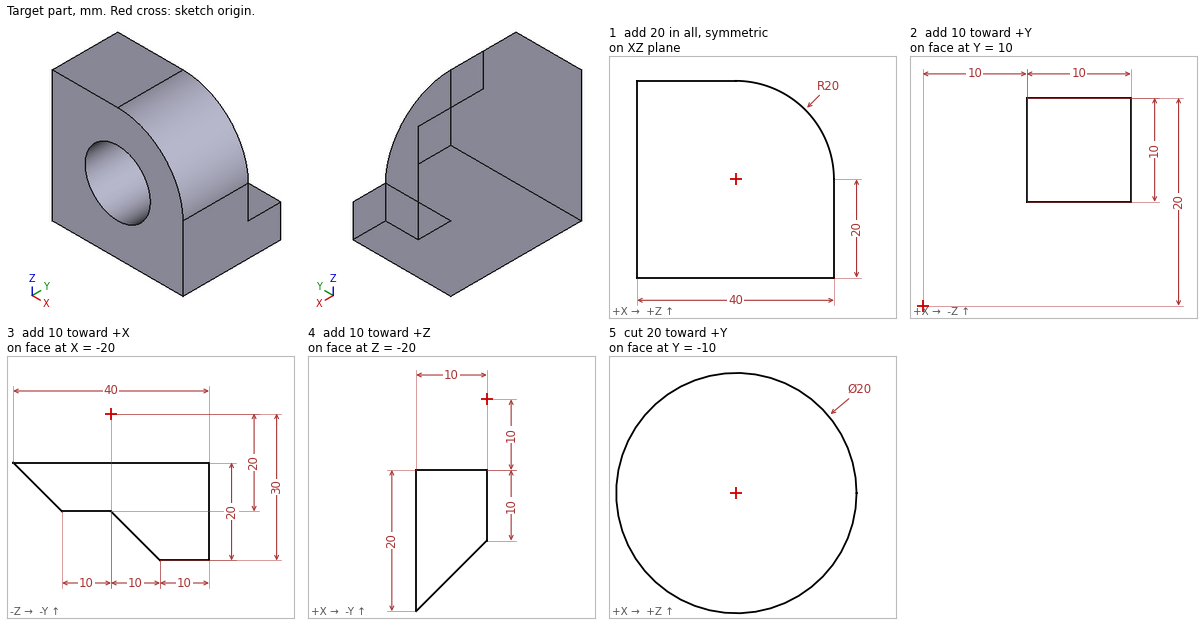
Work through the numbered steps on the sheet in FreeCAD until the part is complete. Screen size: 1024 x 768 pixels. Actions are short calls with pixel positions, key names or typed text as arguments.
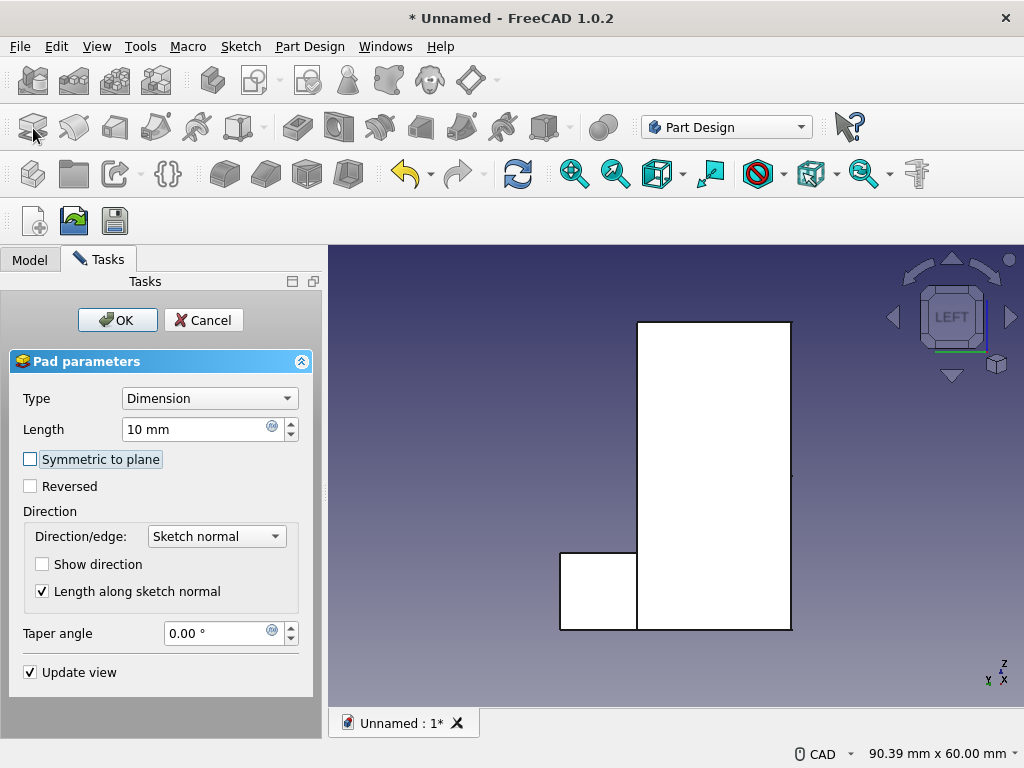
click(31, 486)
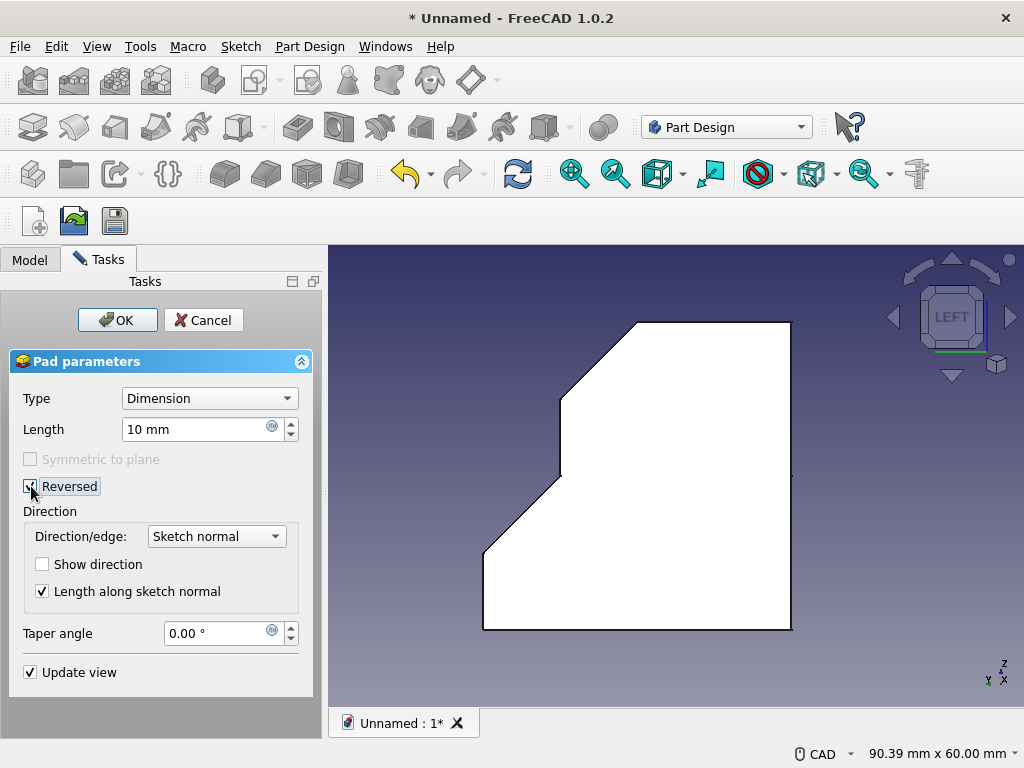
click(118, 320)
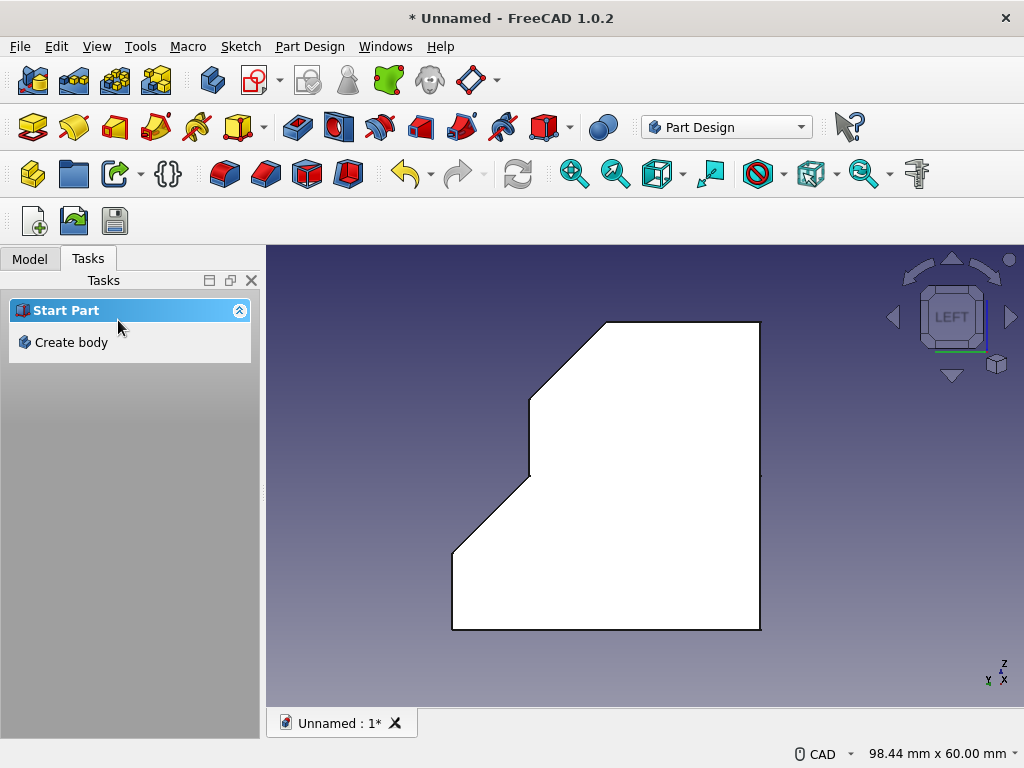
key(5)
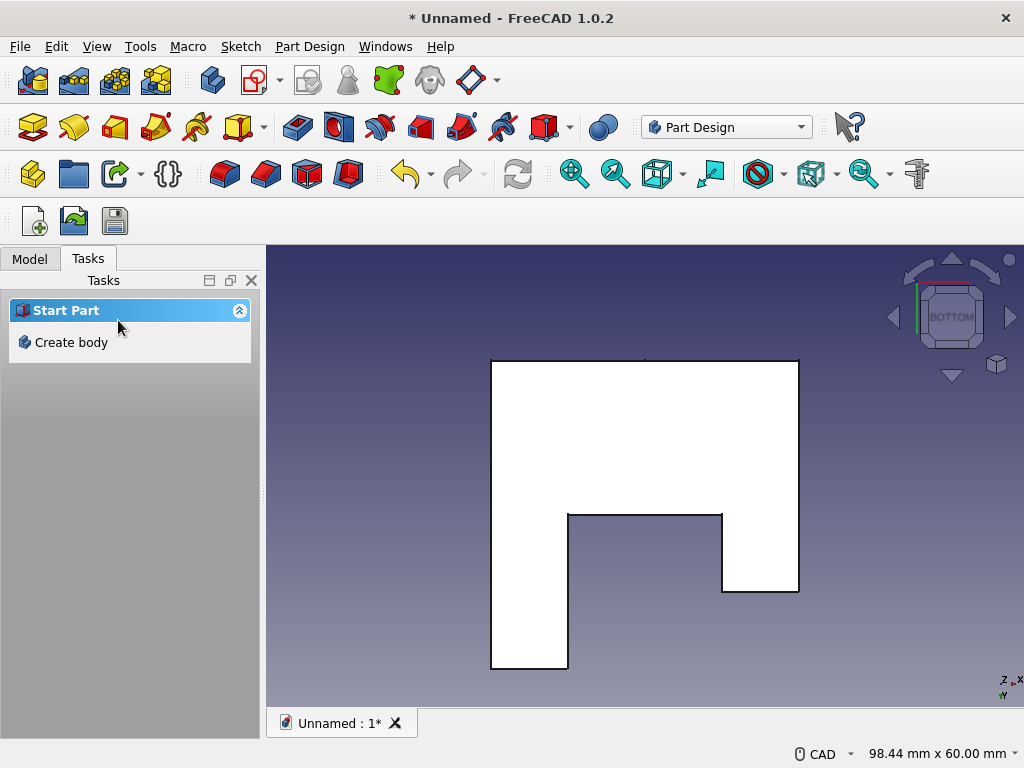
click(733, 426)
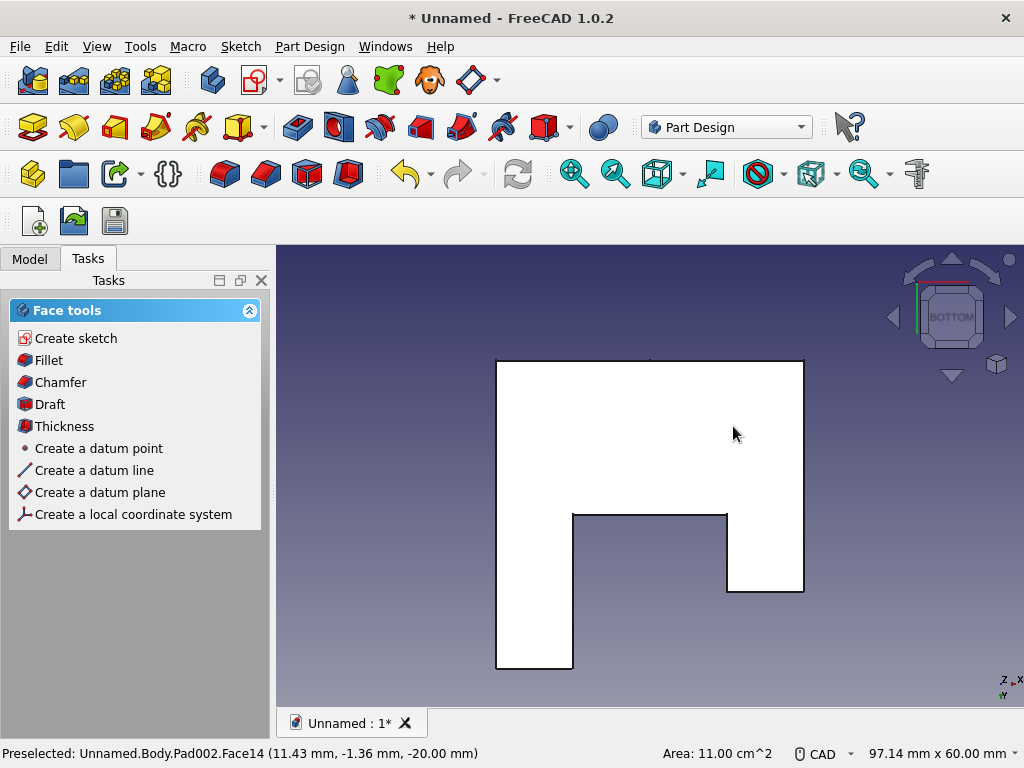
click(254, 80)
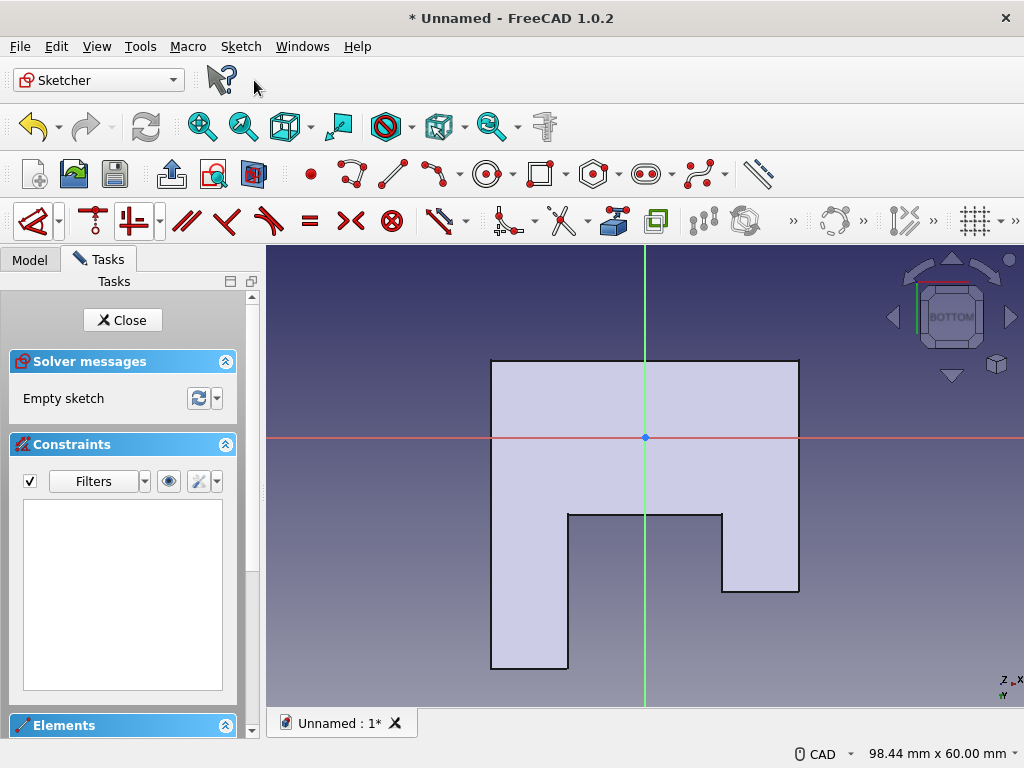
scroll(441, 273, down, 1)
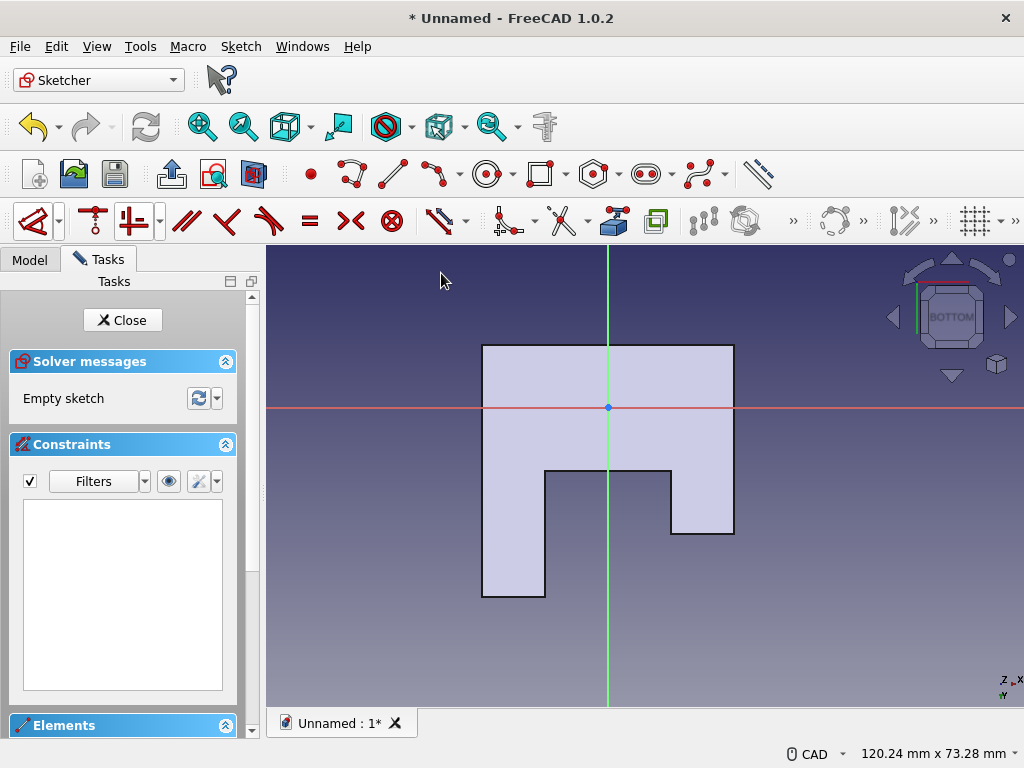
scroll(577, 556, up, 2)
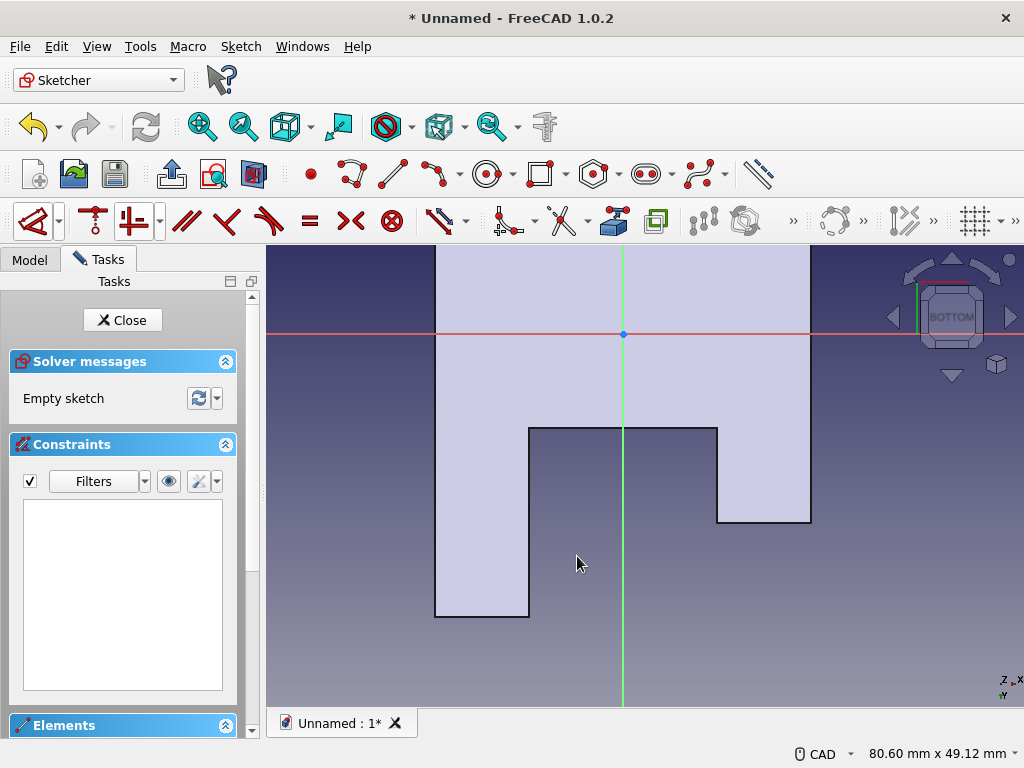
click(352, 174)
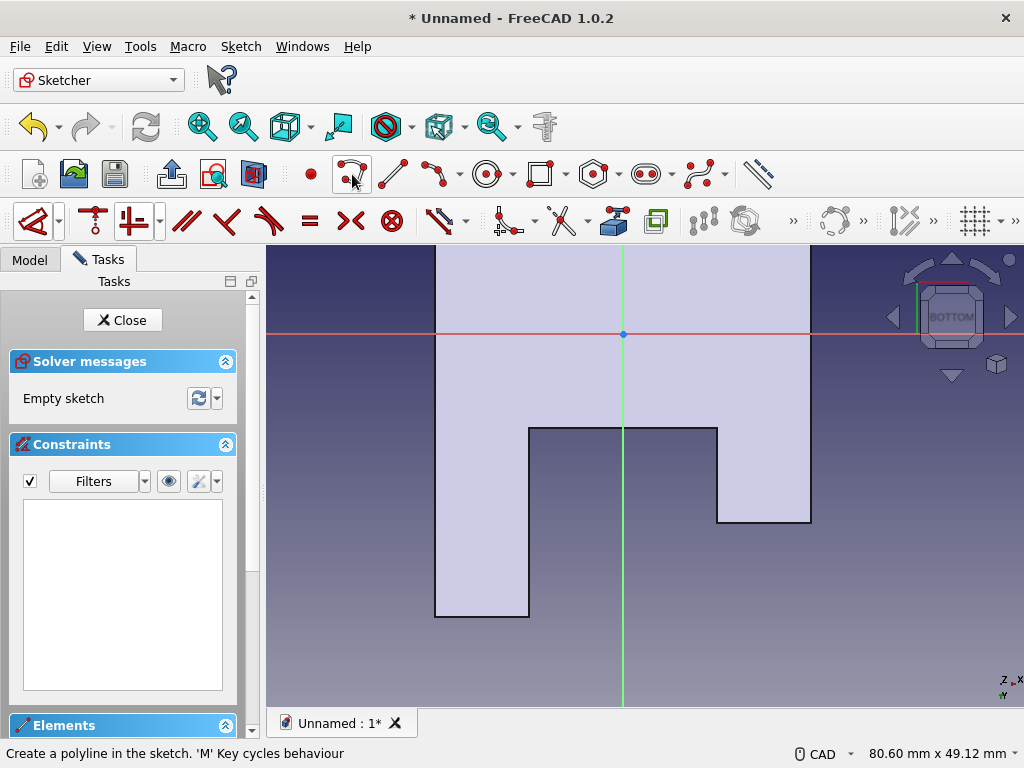
click(623, 428)
click(529, 428)
click(529, 617)
click(614, 523)
click(623, 429)
key(Escape)
key(Escape)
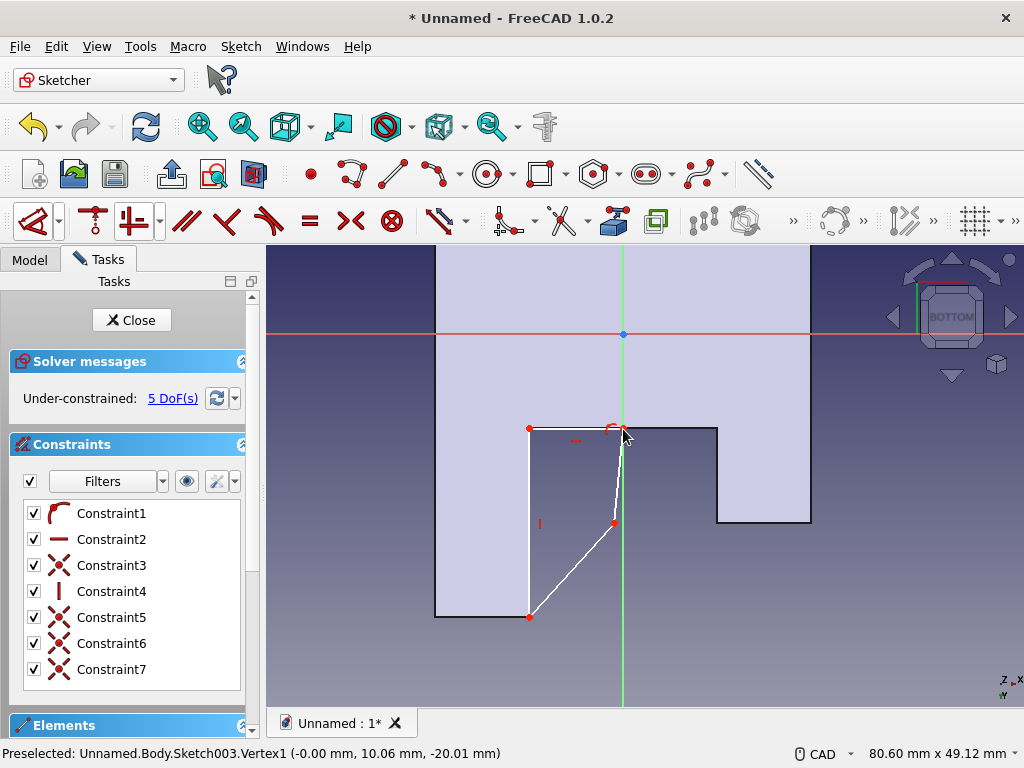
click(620, 457)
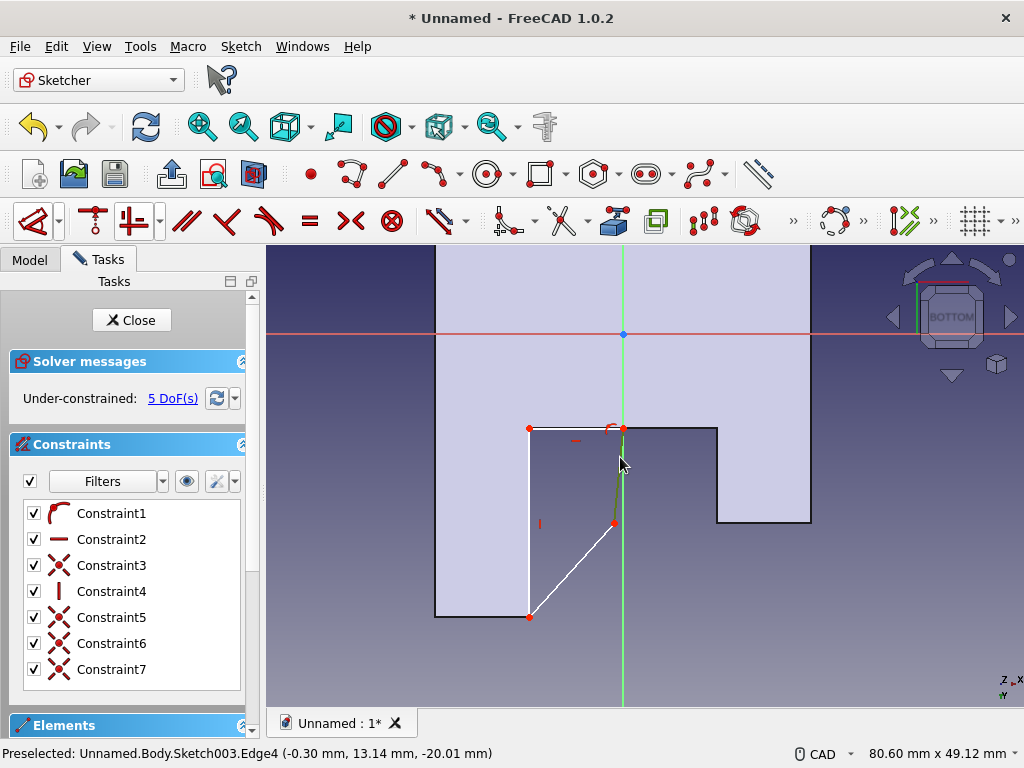
click(160, 222)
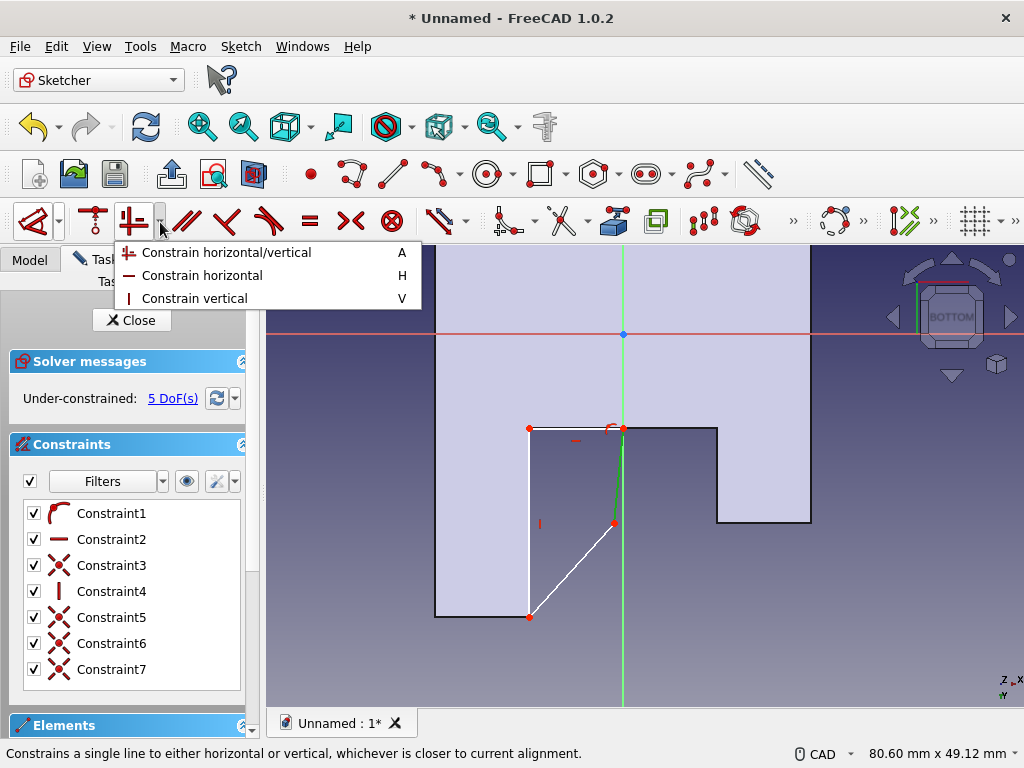
click(268, 298)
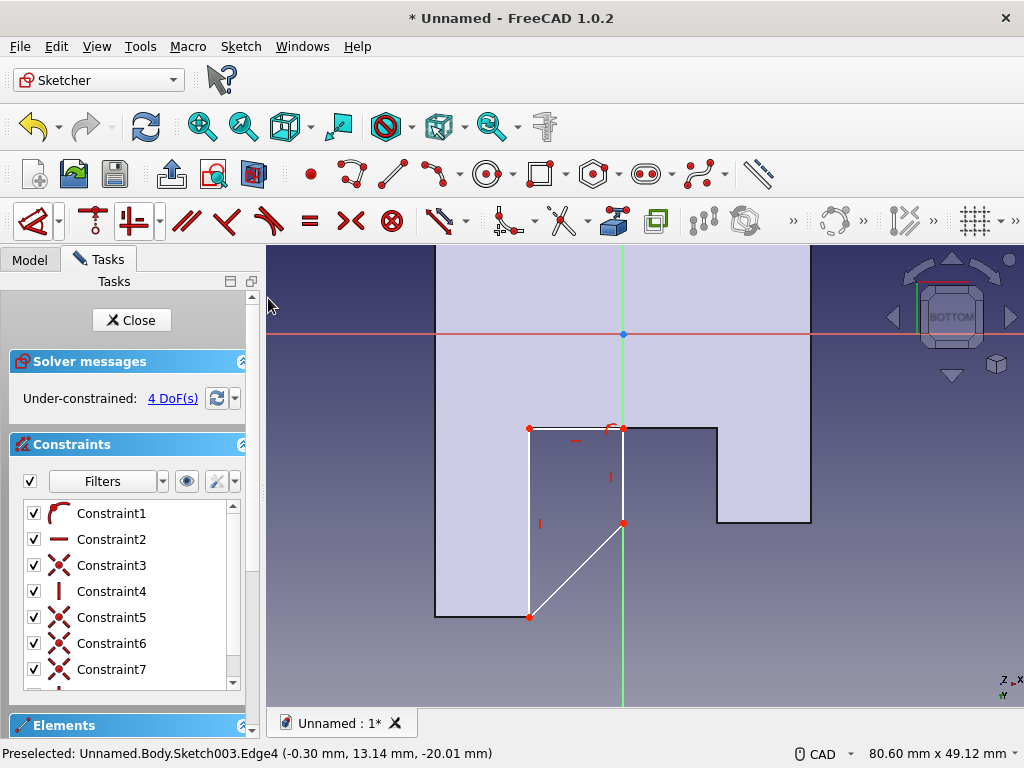
click(595, 429)